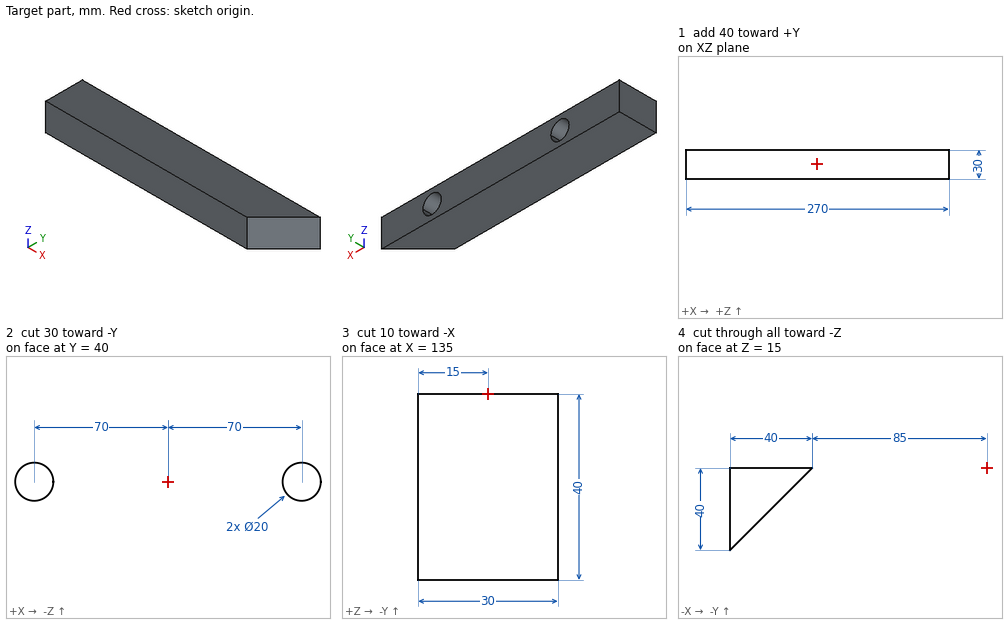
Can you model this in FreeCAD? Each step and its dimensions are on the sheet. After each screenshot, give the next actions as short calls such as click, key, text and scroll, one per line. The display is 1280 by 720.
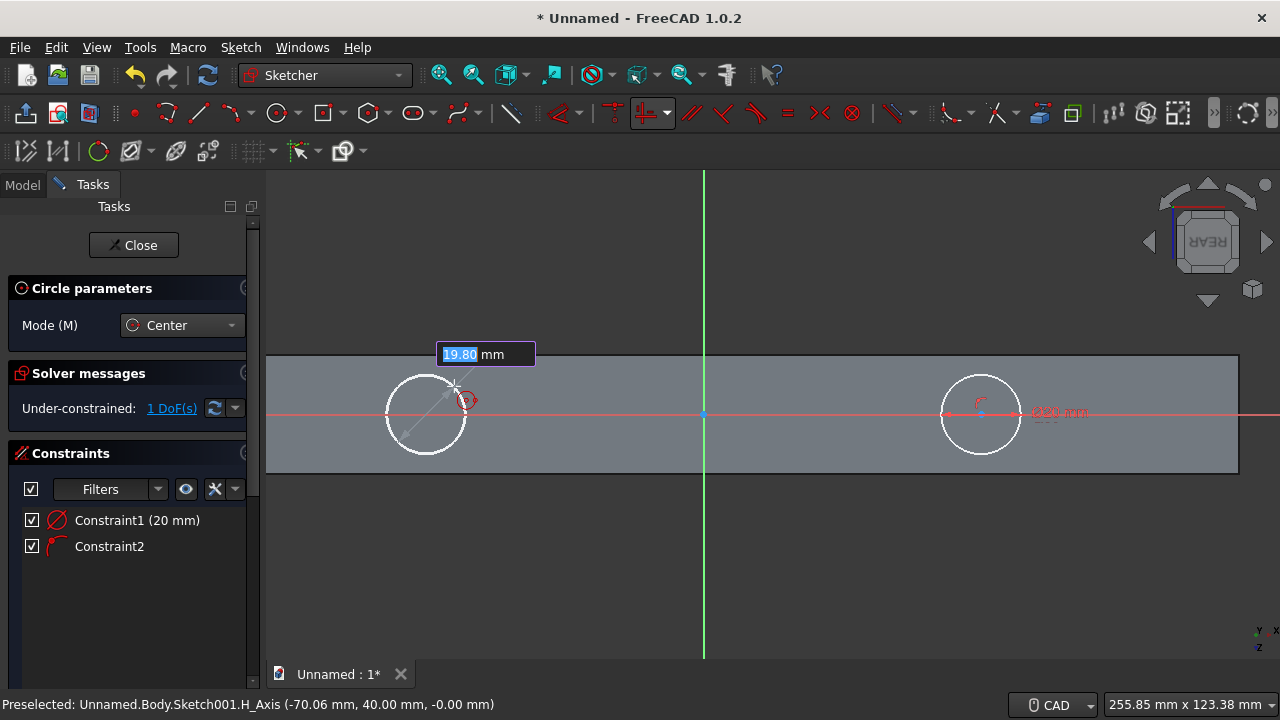
text(20)
key(Return)
key(Escape)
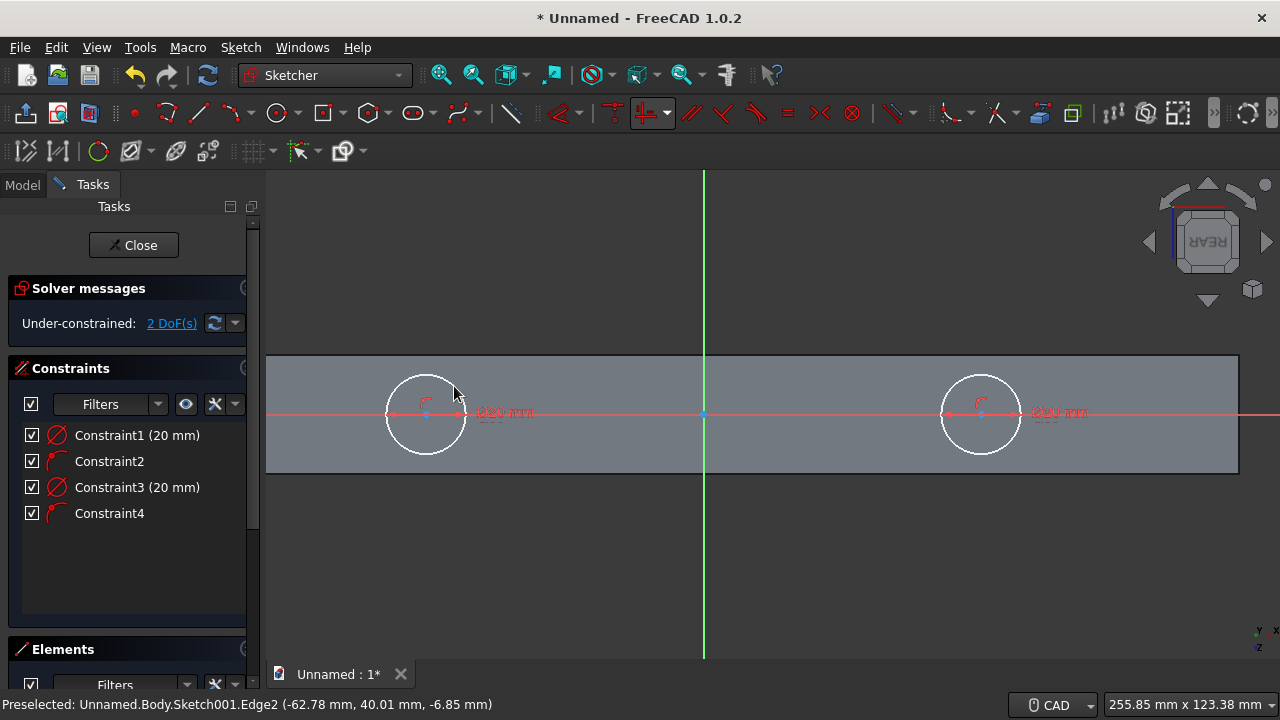
click(558, 114)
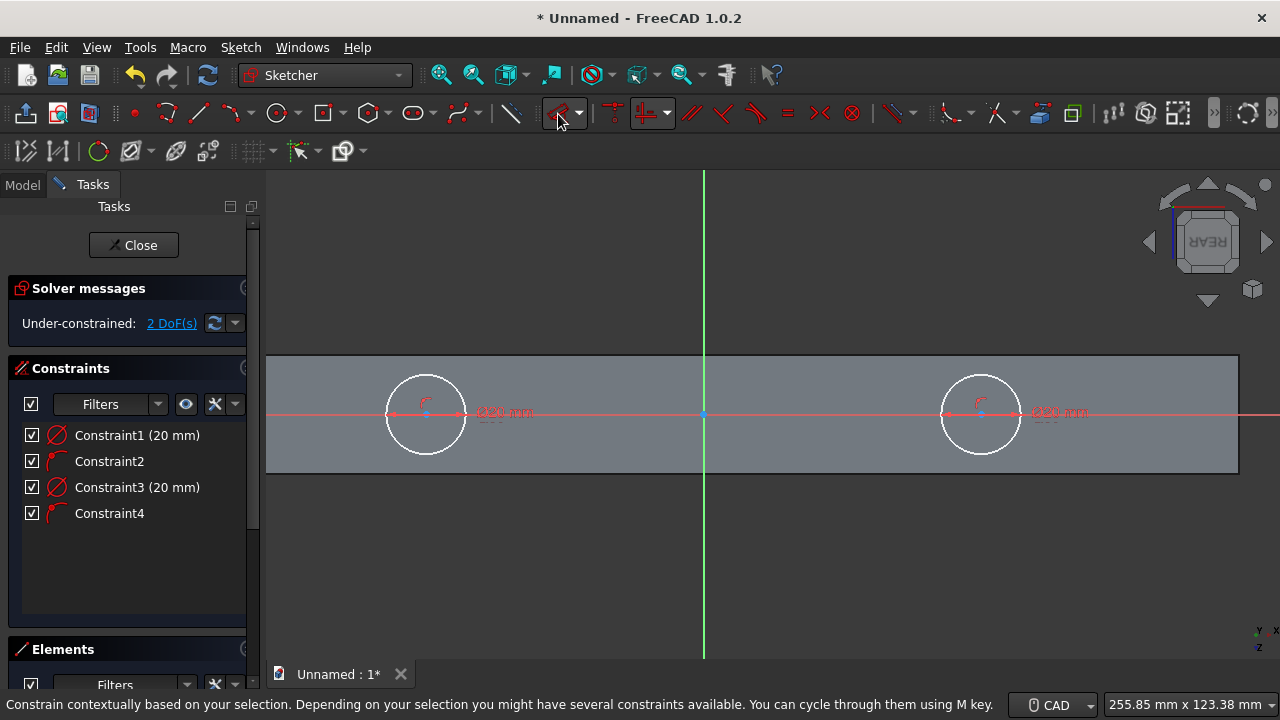
click(981, 414)
click(842, 448)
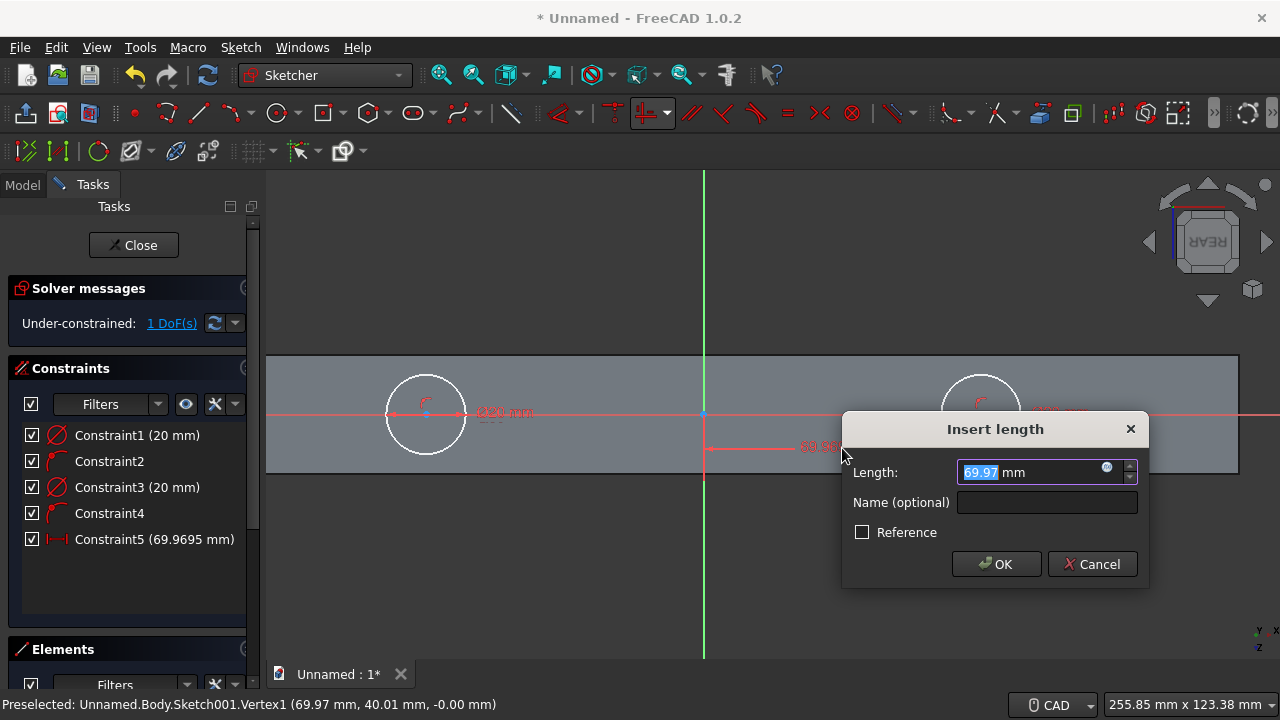
text(70)
key(Return)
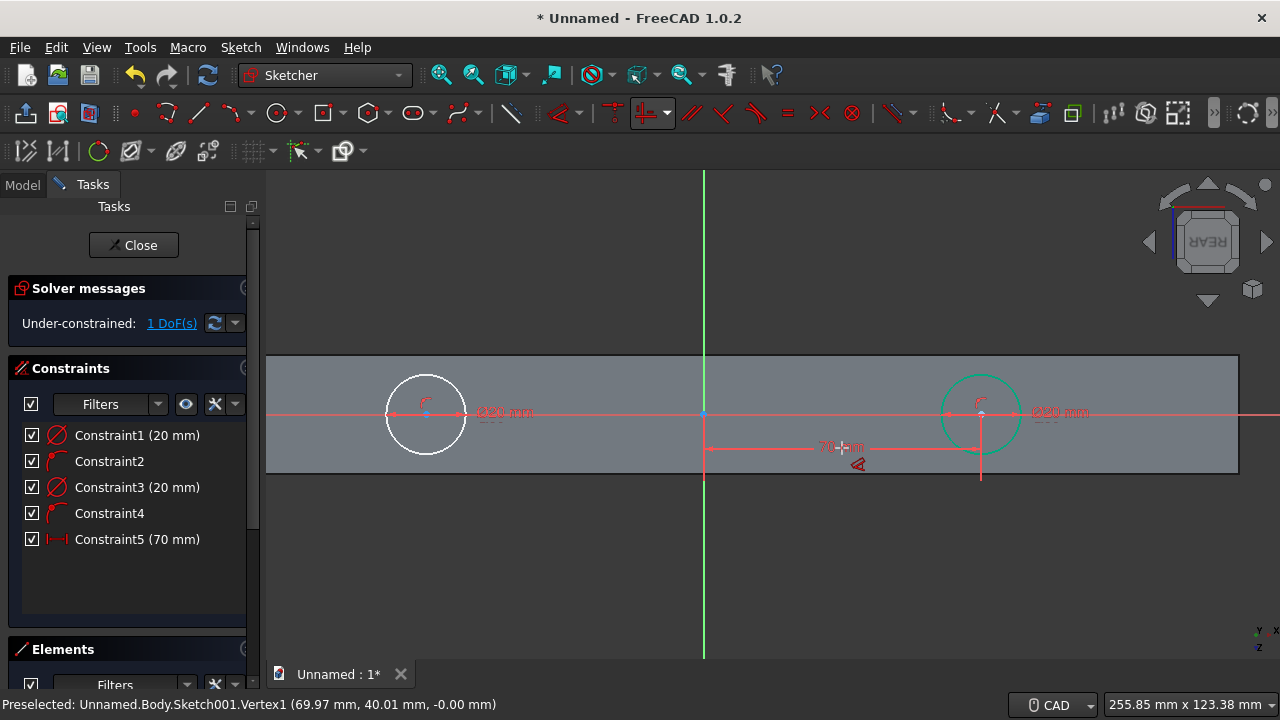
click(426, 414)
click(565, 448)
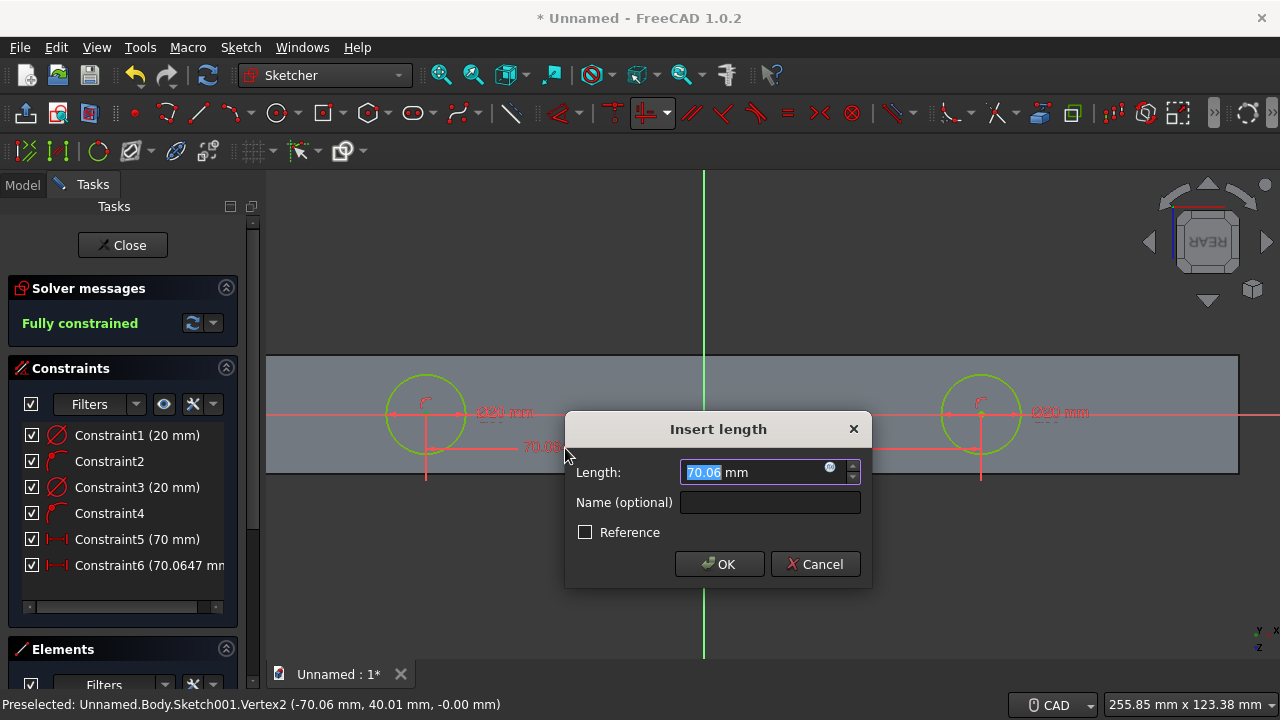
text(70)
key(Return)
key(Escape)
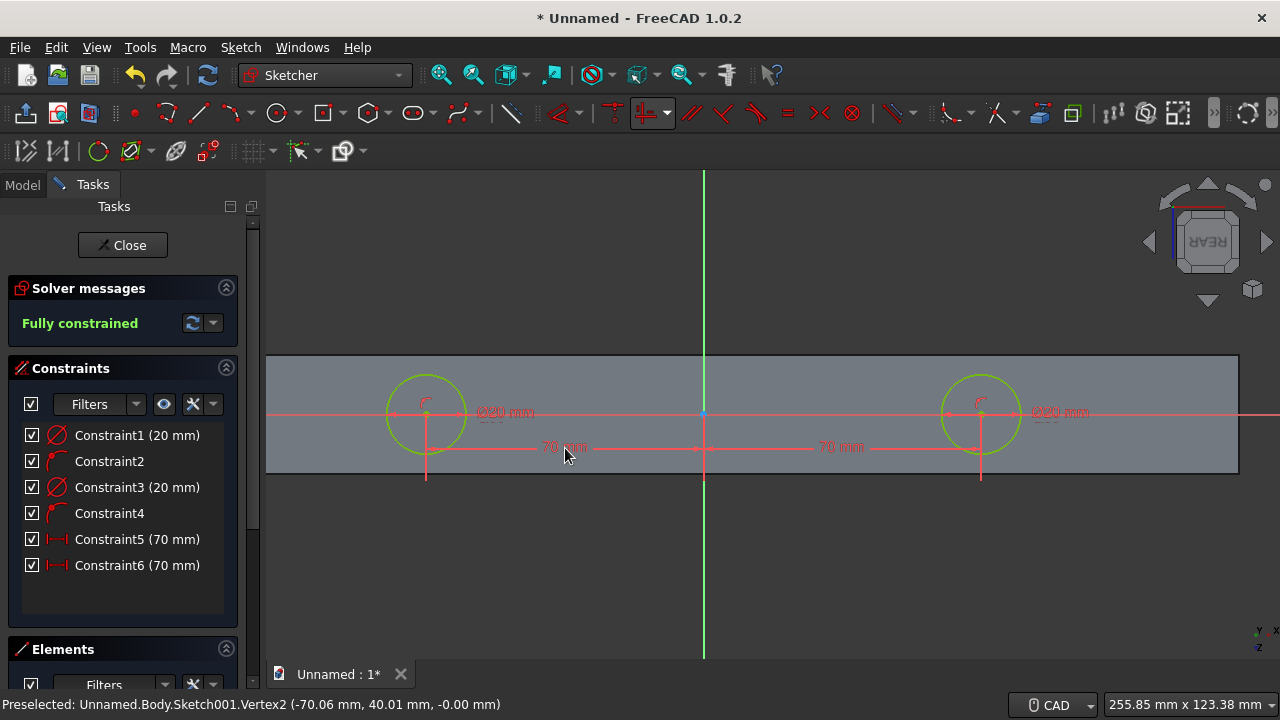
click(123, 245)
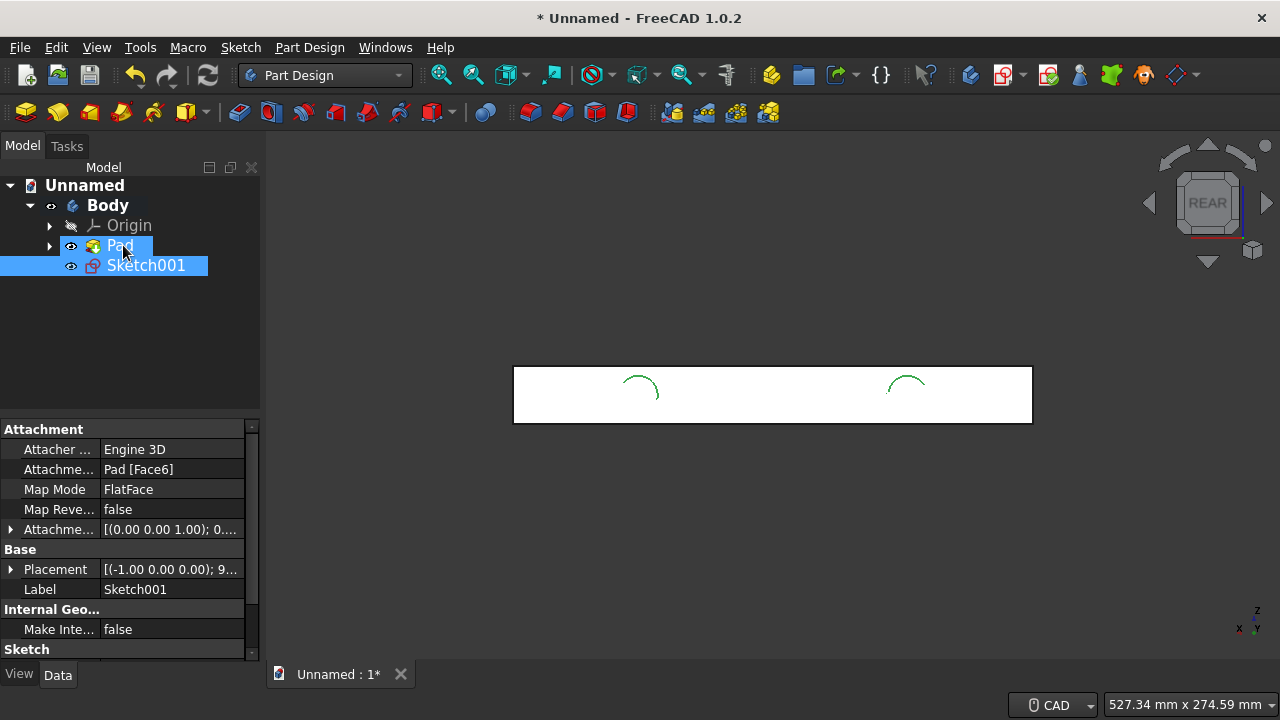
click(240, 112)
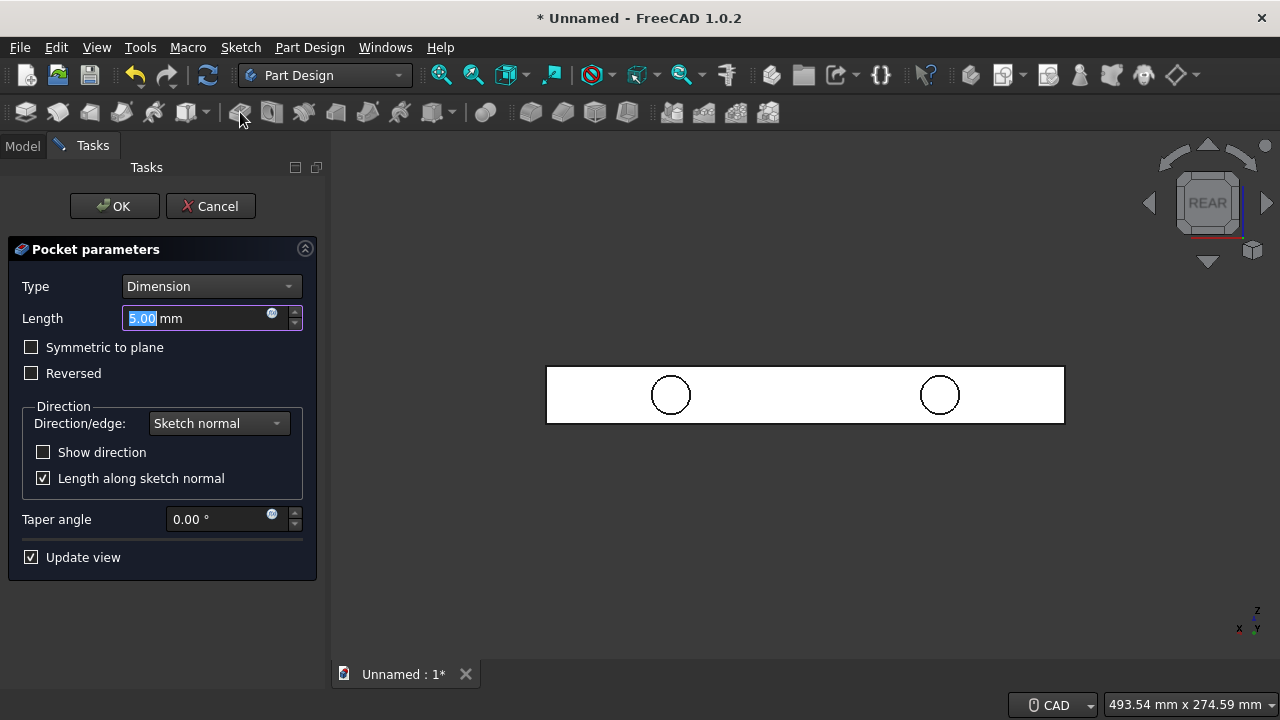
text(30)
key(Tab)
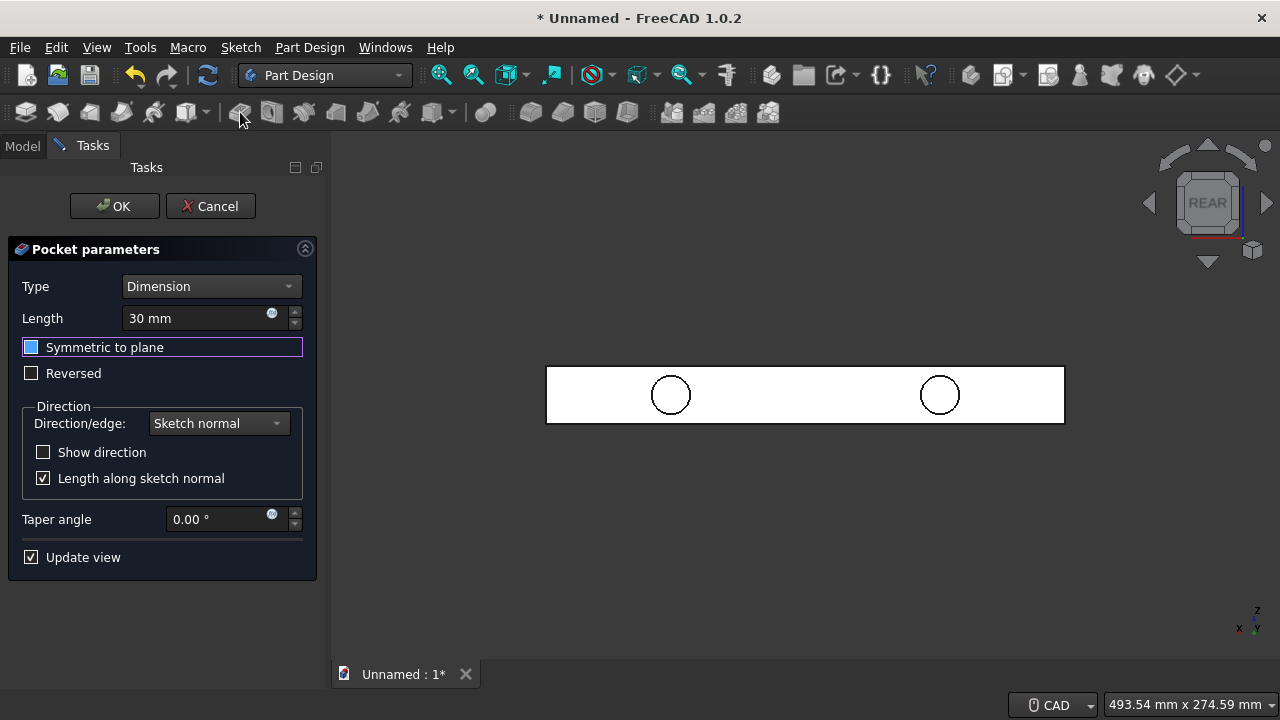
click(115, 206)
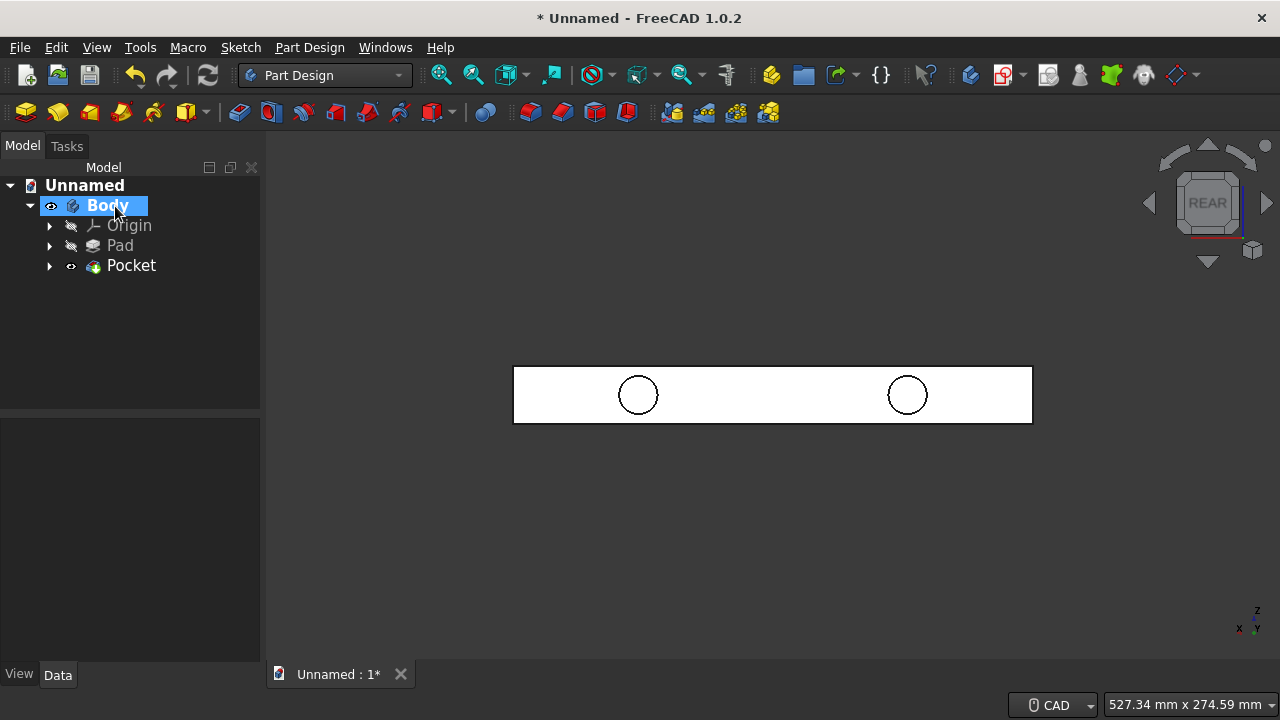
key(0)